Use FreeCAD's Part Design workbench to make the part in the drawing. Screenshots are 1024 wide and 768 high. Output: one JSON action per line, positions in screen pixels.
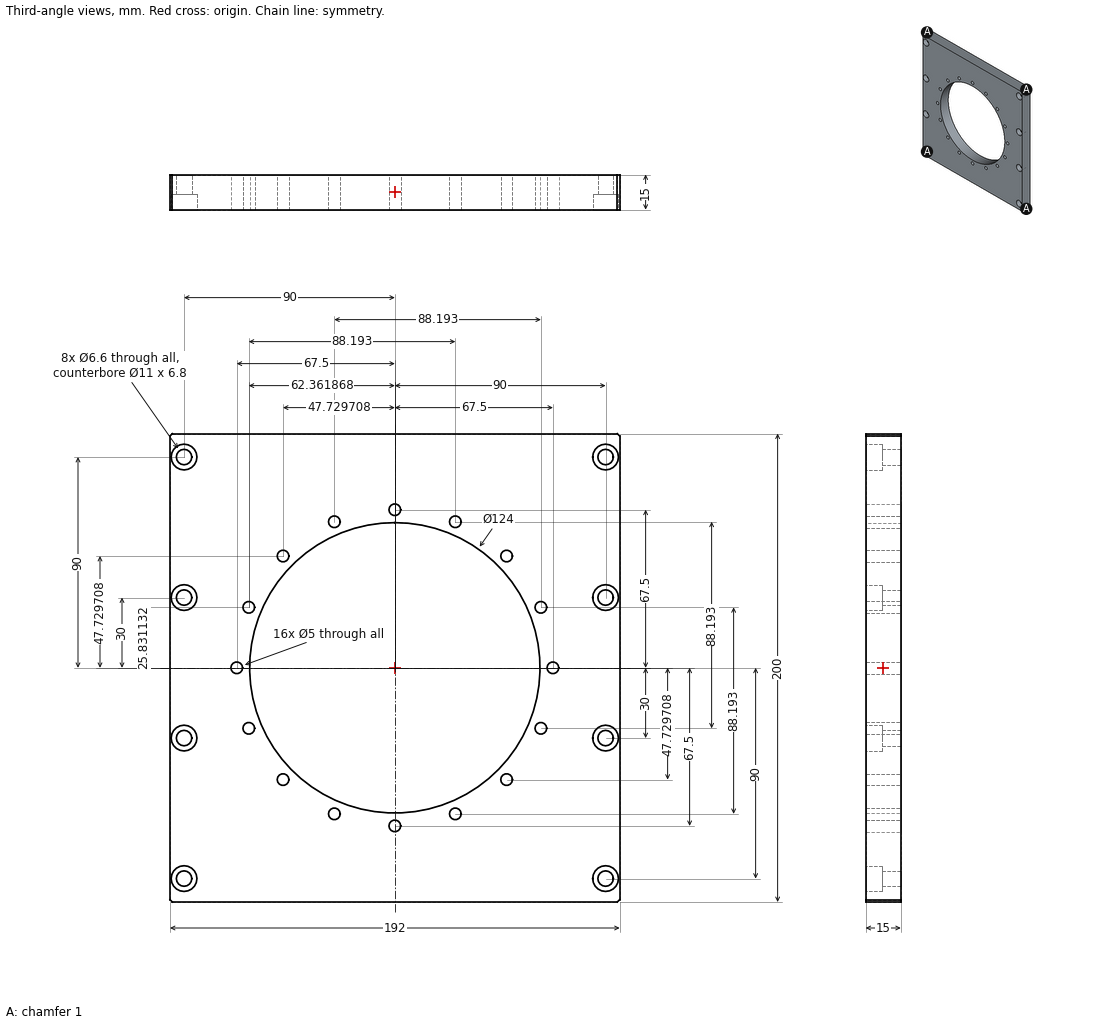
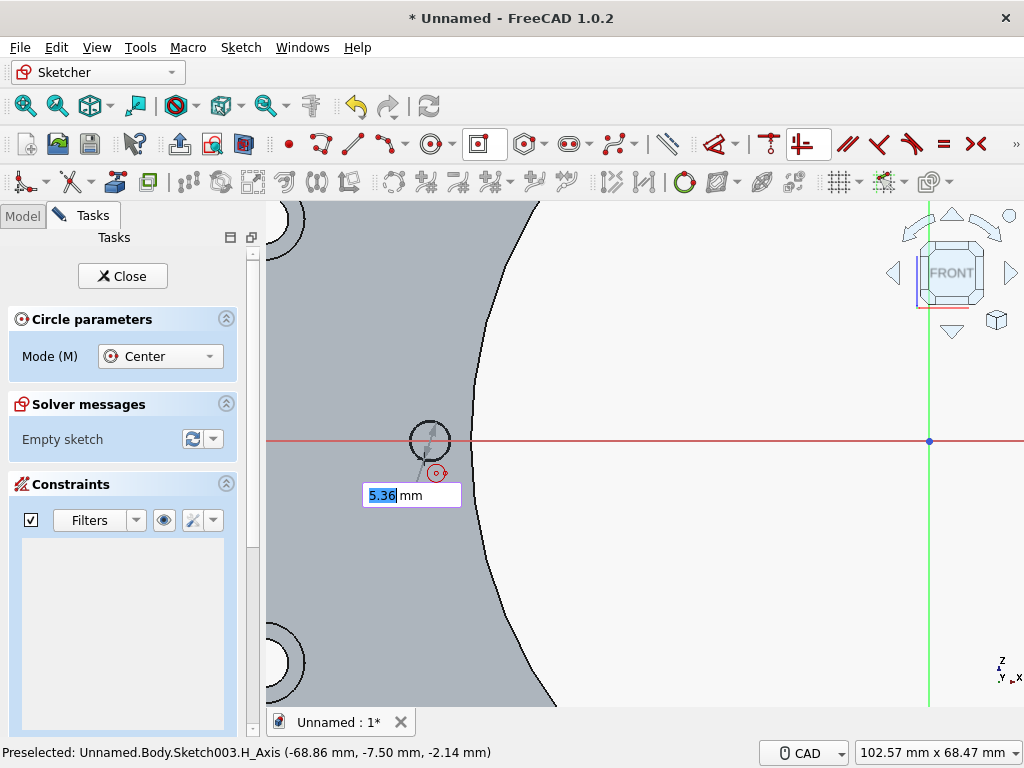
{"action": "type", "text": "5"}
{"action": "key", "text": "Return"}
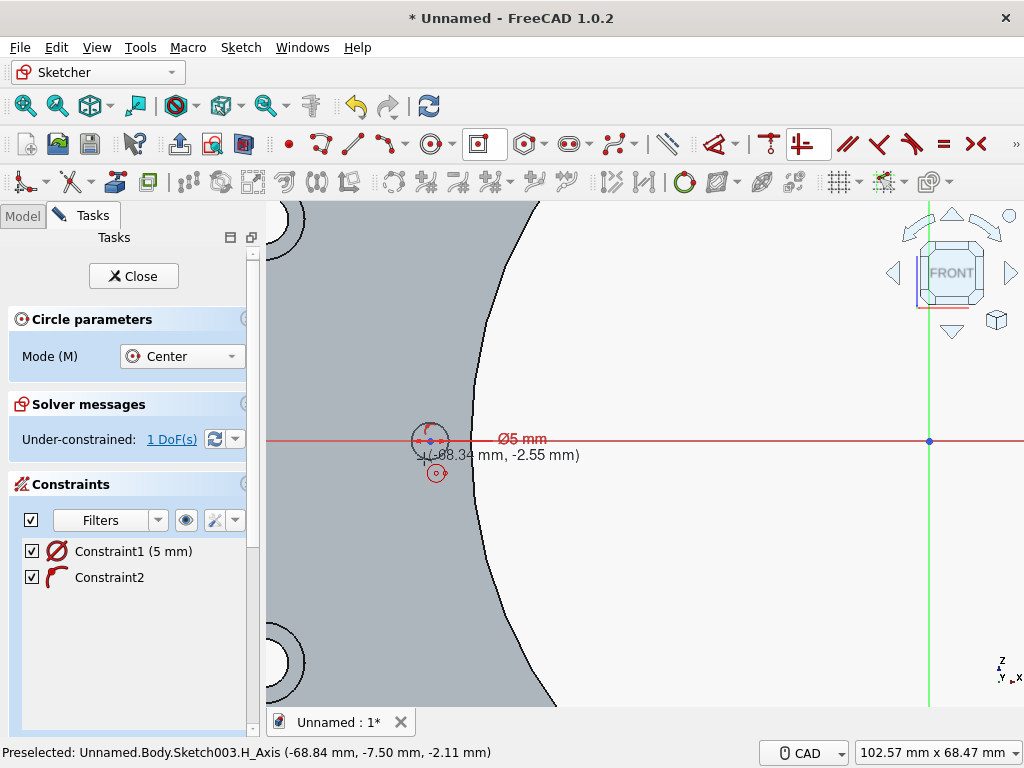
{"action": "scroll", "coordinate": [468, 250], "scroll_direction": "up", "scroll_amount": 2}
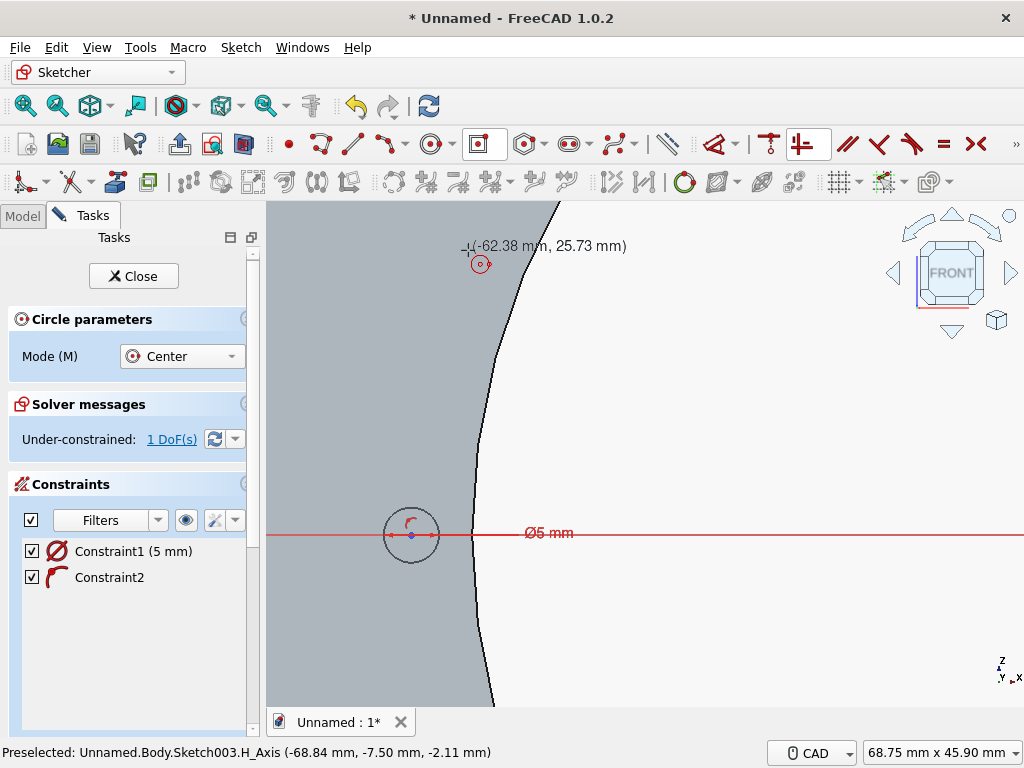
{"action": "scroll", "coordinate": [430, 433], "scroll_direction": "down", "scroll_amount": 8}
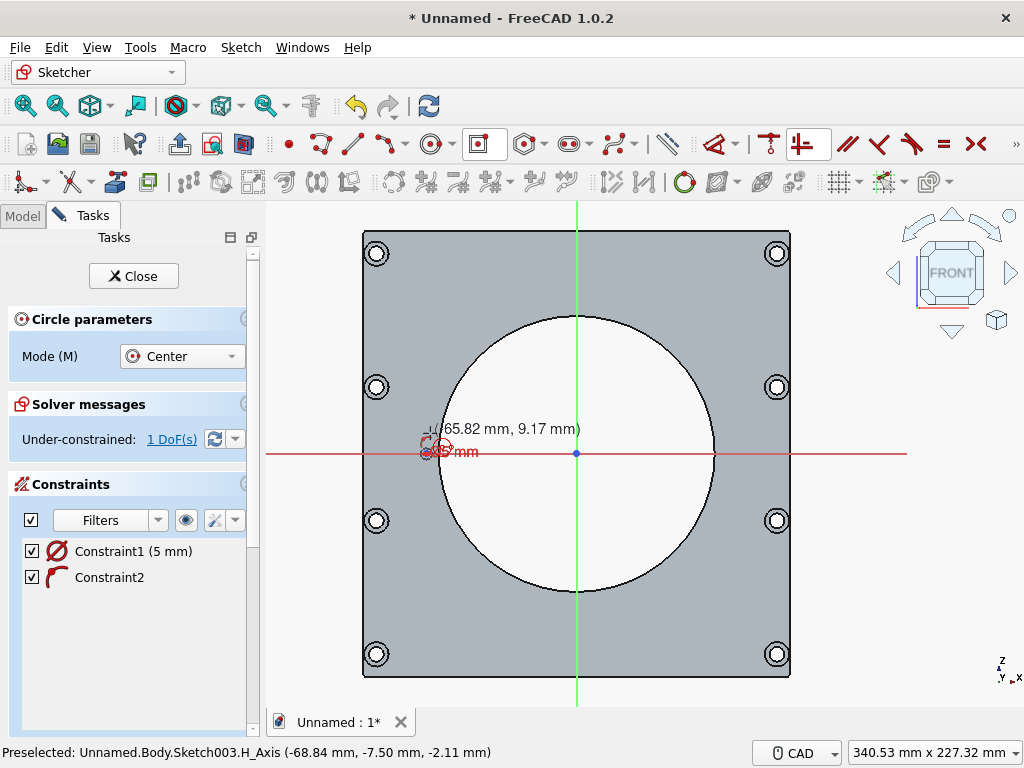
{"action": "left_click", "coordinate": [438, 396]}
{"action": "mouse_move", "coordinate": [442, 393]}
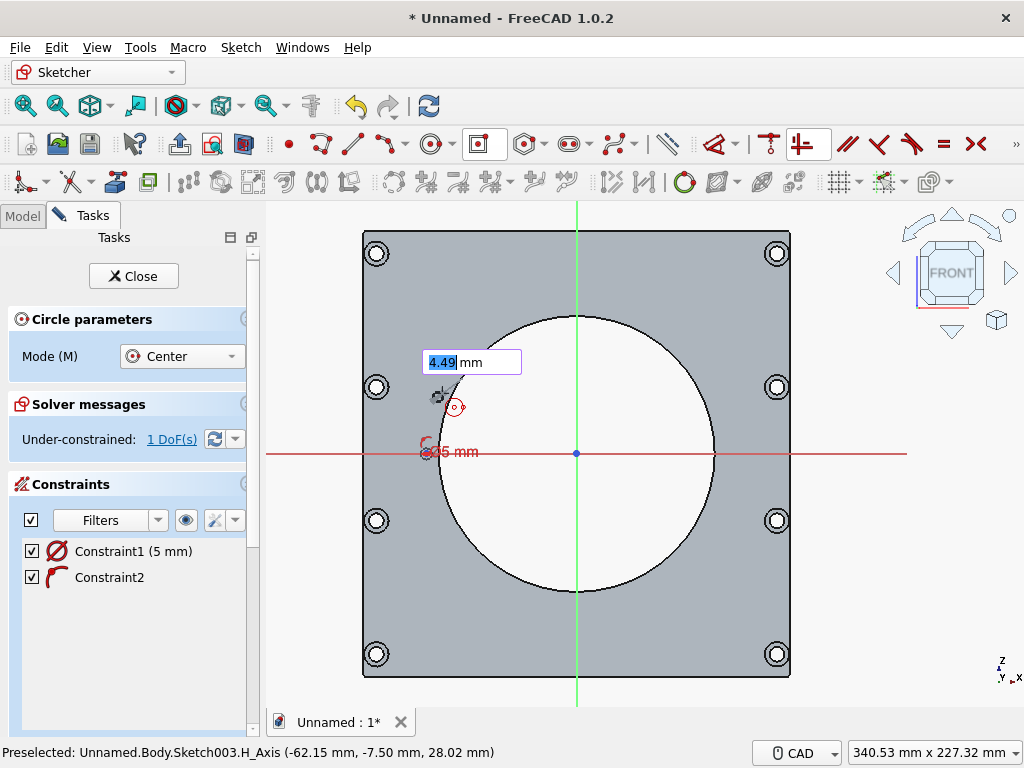
{"action": "type", "text": "5"}
{"action": "key", "text": "Return"}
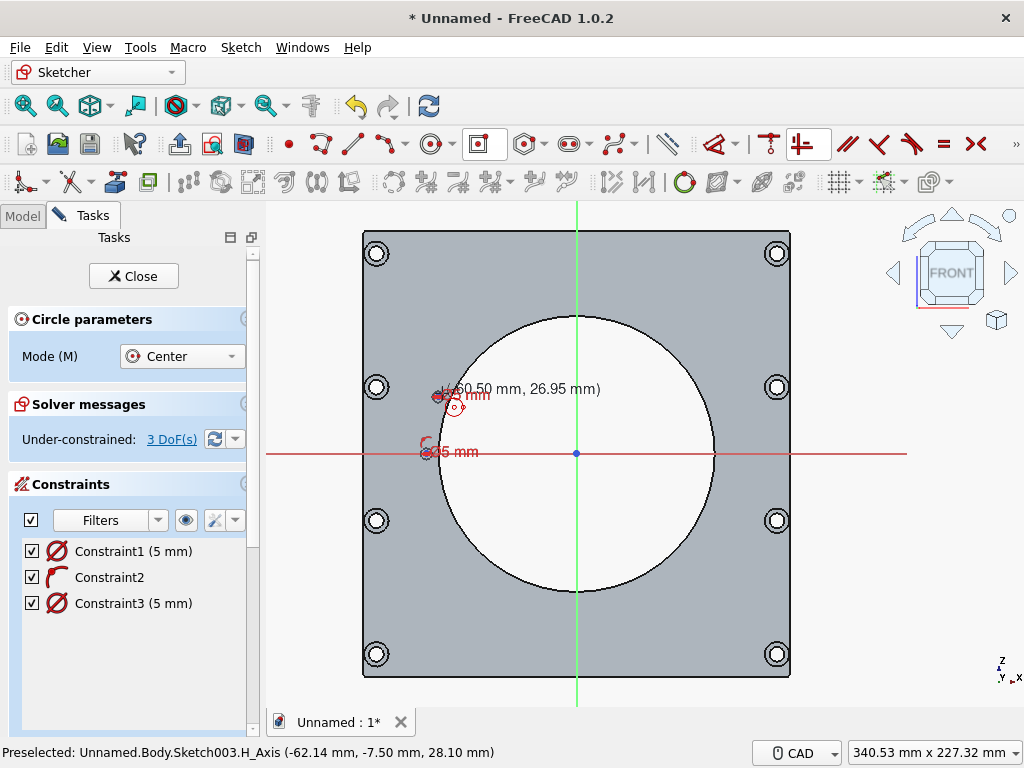
{"action": "scroll", "coordinate": [470, 348], "scroll_direction": "up", "scroll_amount": 8}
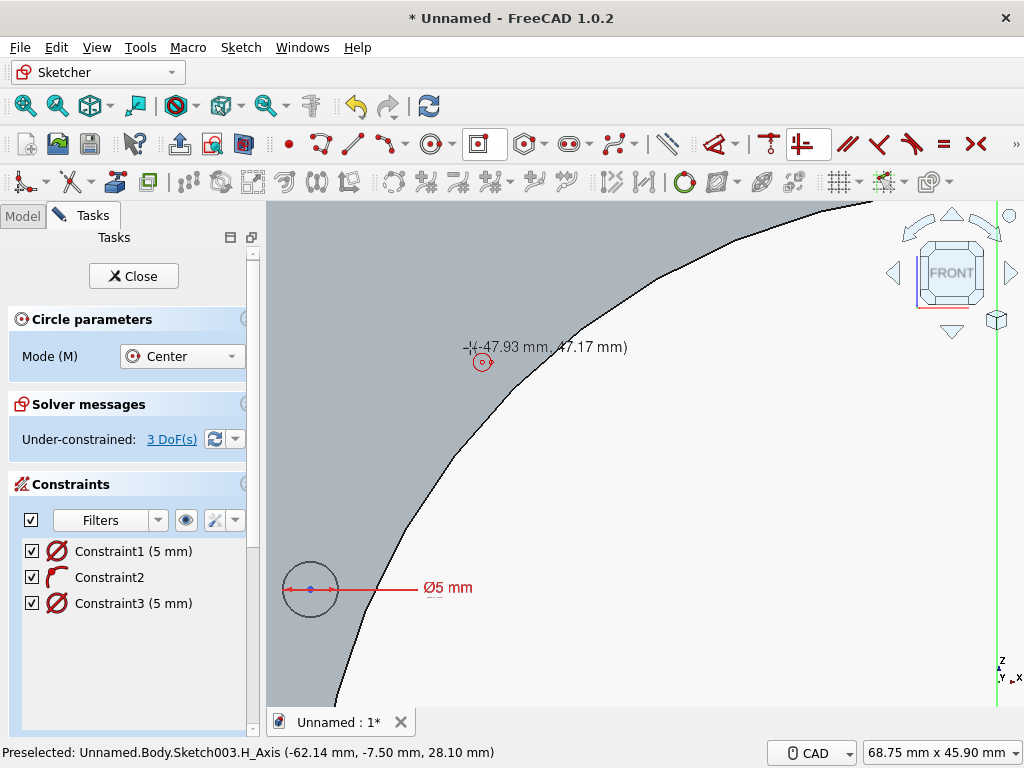
{"action": "scroll", "coordinate": [470, 348], "scroll_direction": "down", "scroll_amount": 8}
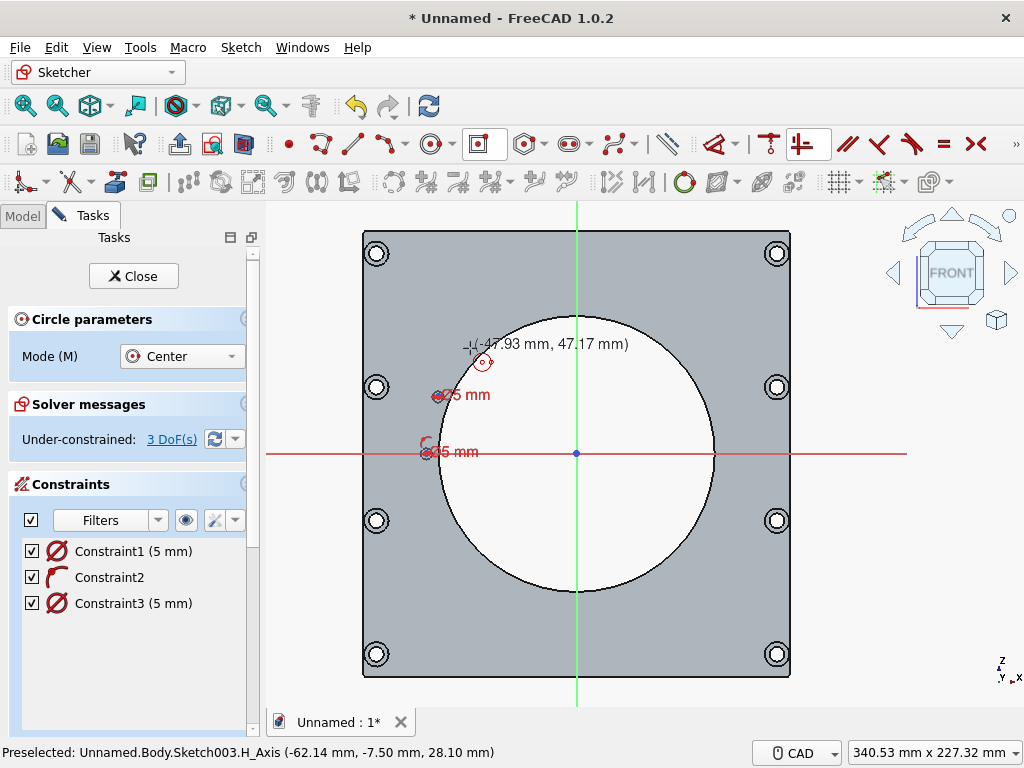
{"action": "left_click", "coordinate": [470, 348]}
{"action": "mouse_move", "coordinate": [474, 344]}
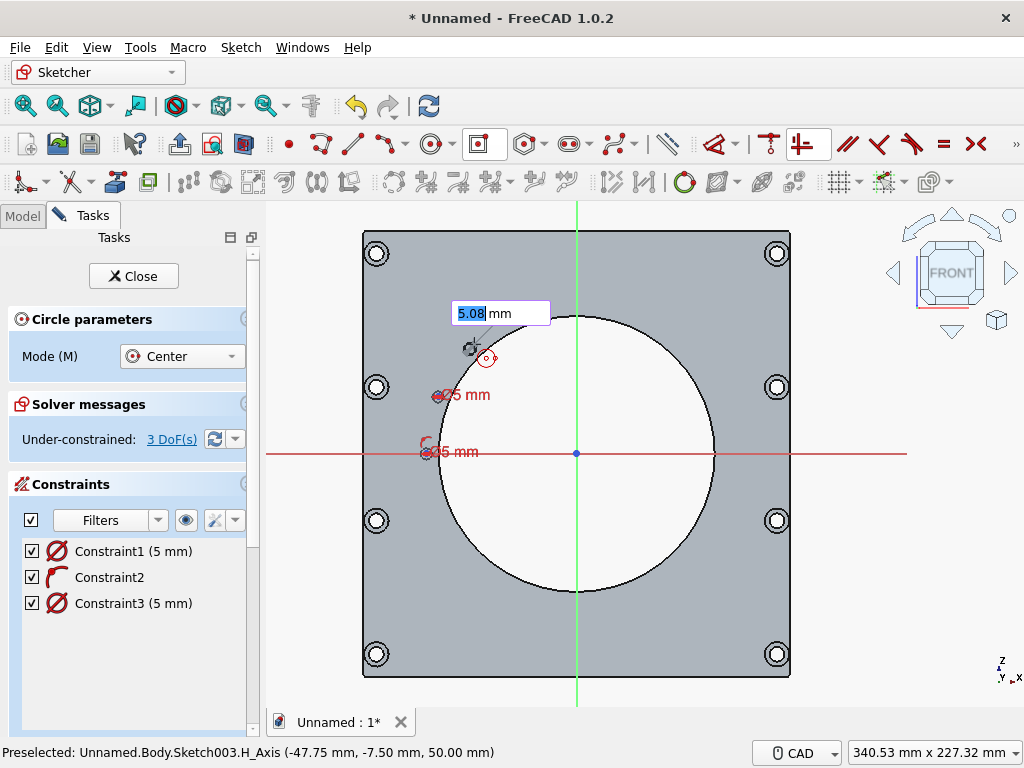
{"action": "type", "text": "5"}
{"action": "key", "text": "Return"}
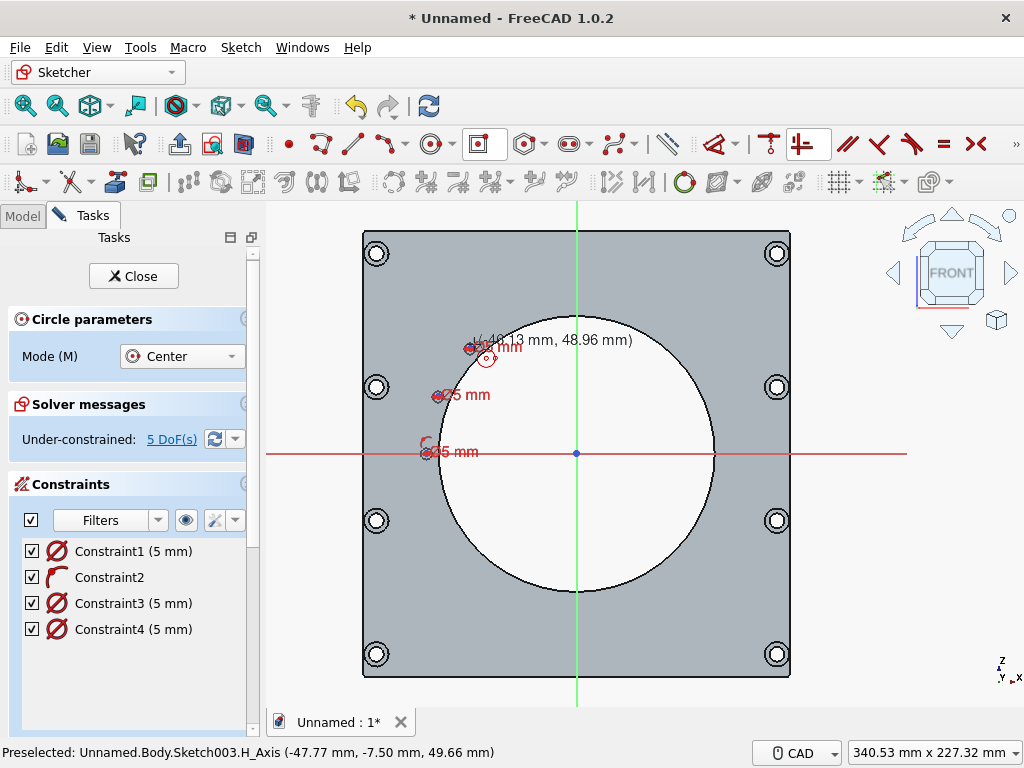
{"action": "scroll", "coordinate": [519, 315], "scroll_direction": "up", "scroll_amount": 8}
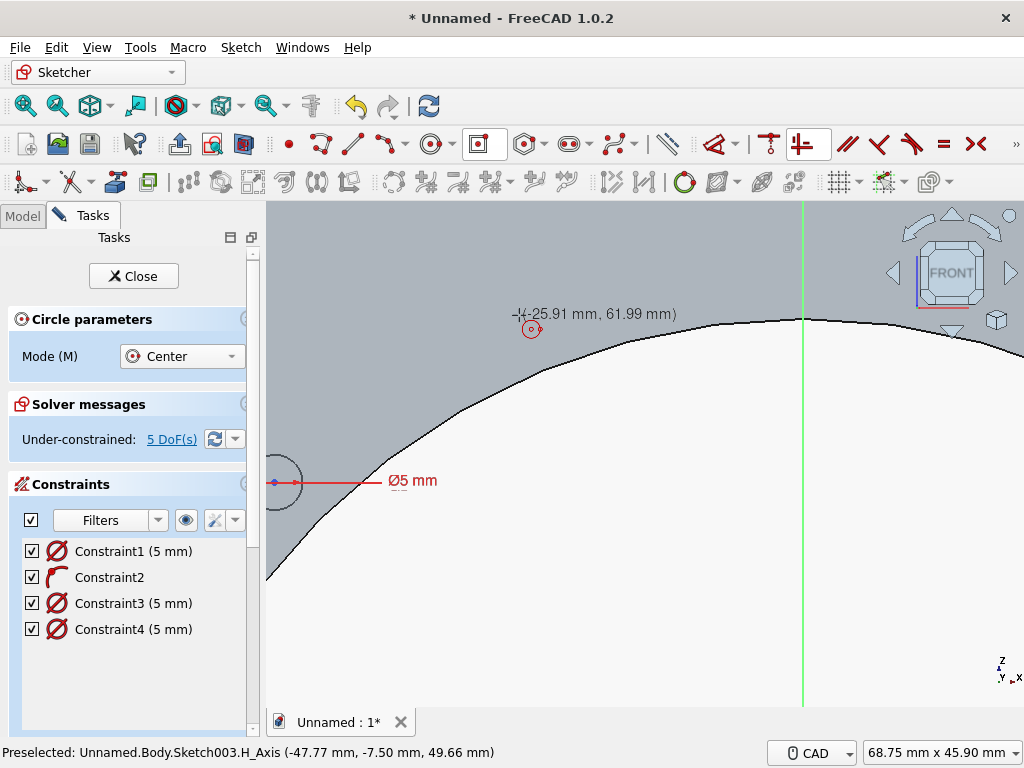
{"action": "scroll", "coordinate": [519, 315], "scroll_direction": "down", "scroll_amount": 8}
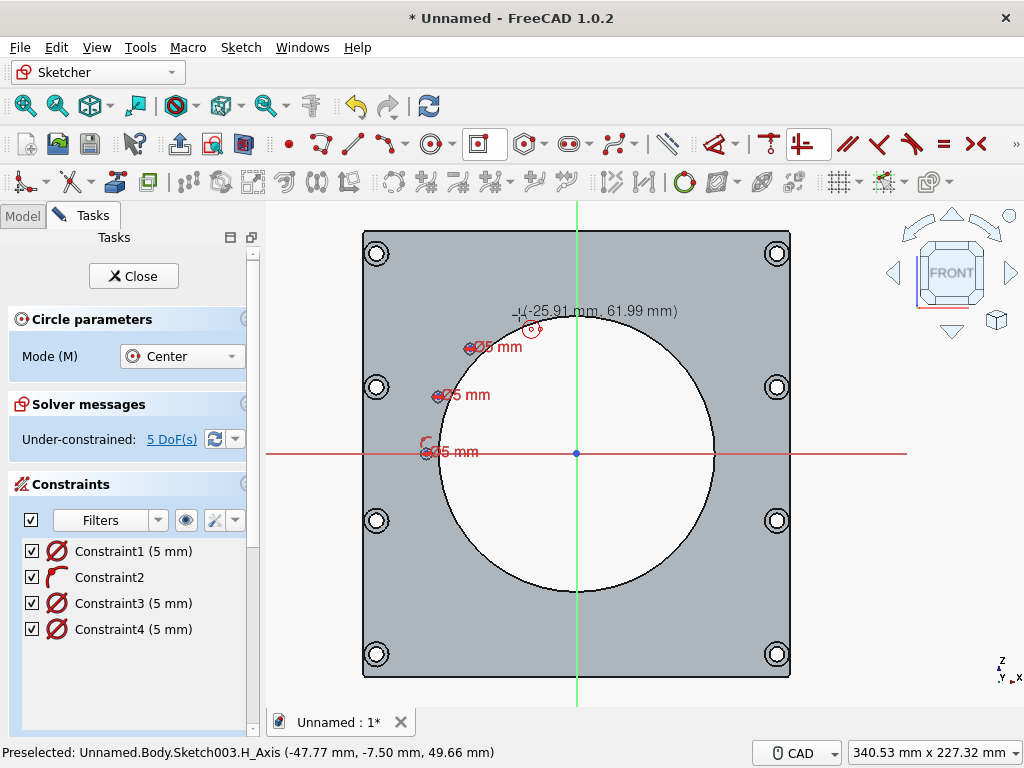
{"action": "left_click", "coordinate": [519, 315]}
{"action": "mouse_move", "coordinate": [523, 311]}